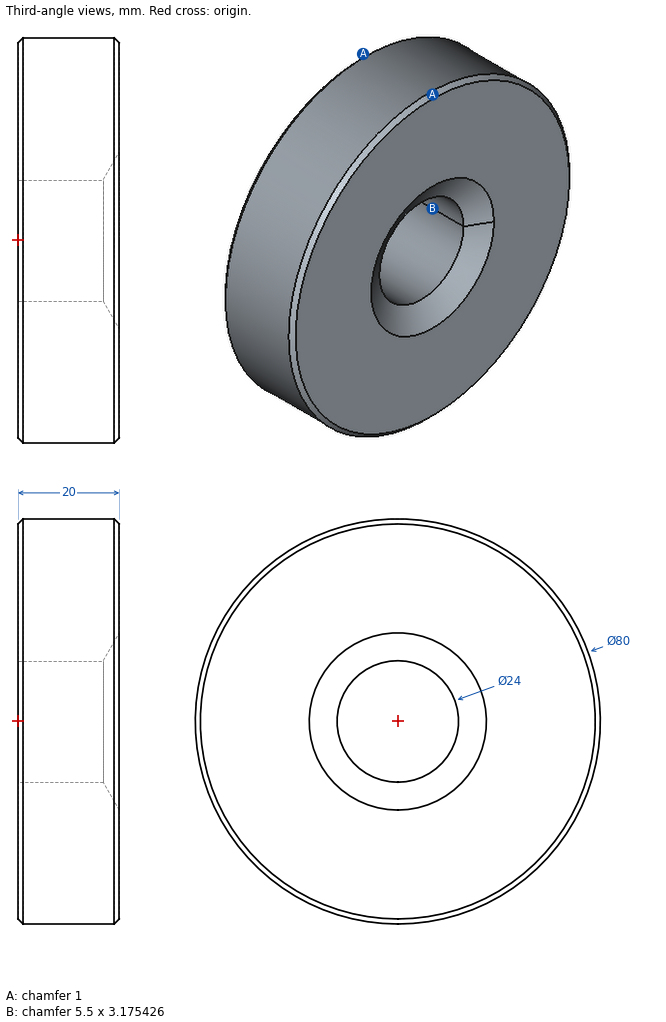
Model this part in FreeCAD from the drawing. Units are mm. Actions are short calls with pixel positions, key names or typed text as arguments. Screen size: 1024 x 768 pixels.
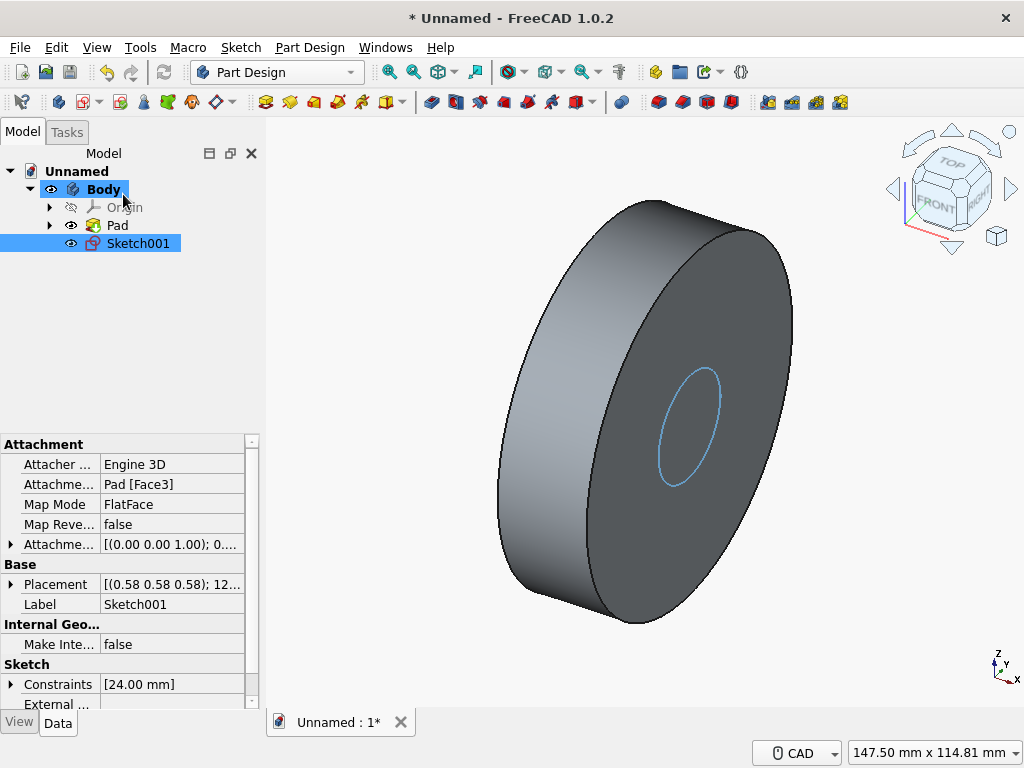
click(432, 102)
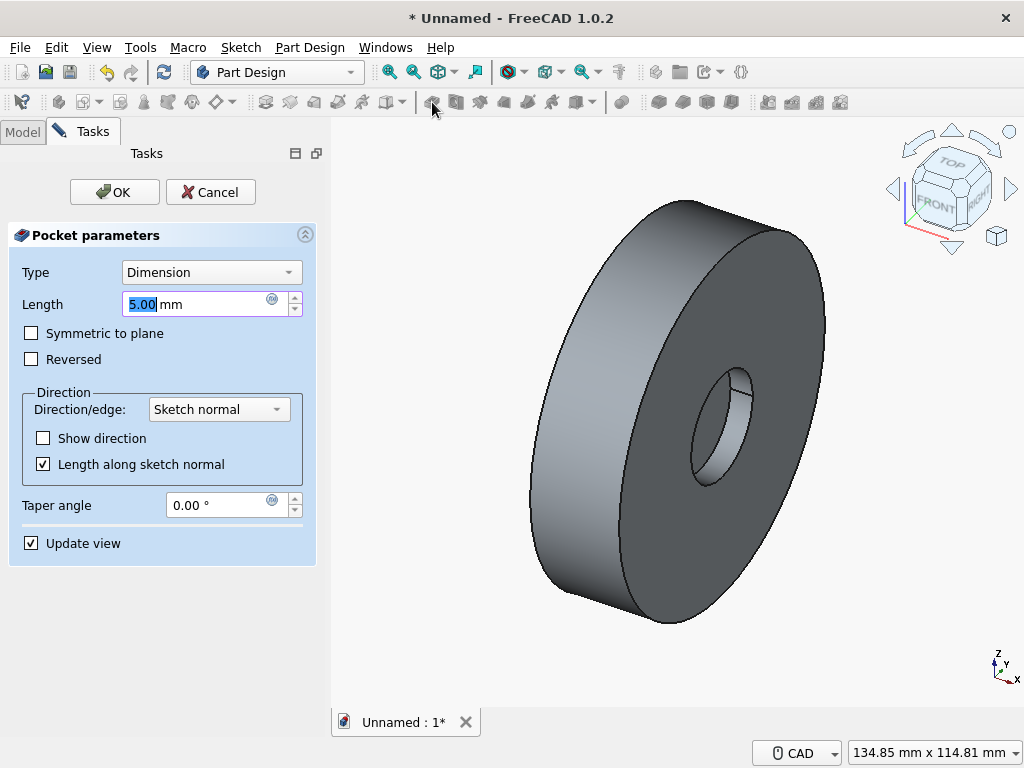
click(212, 272)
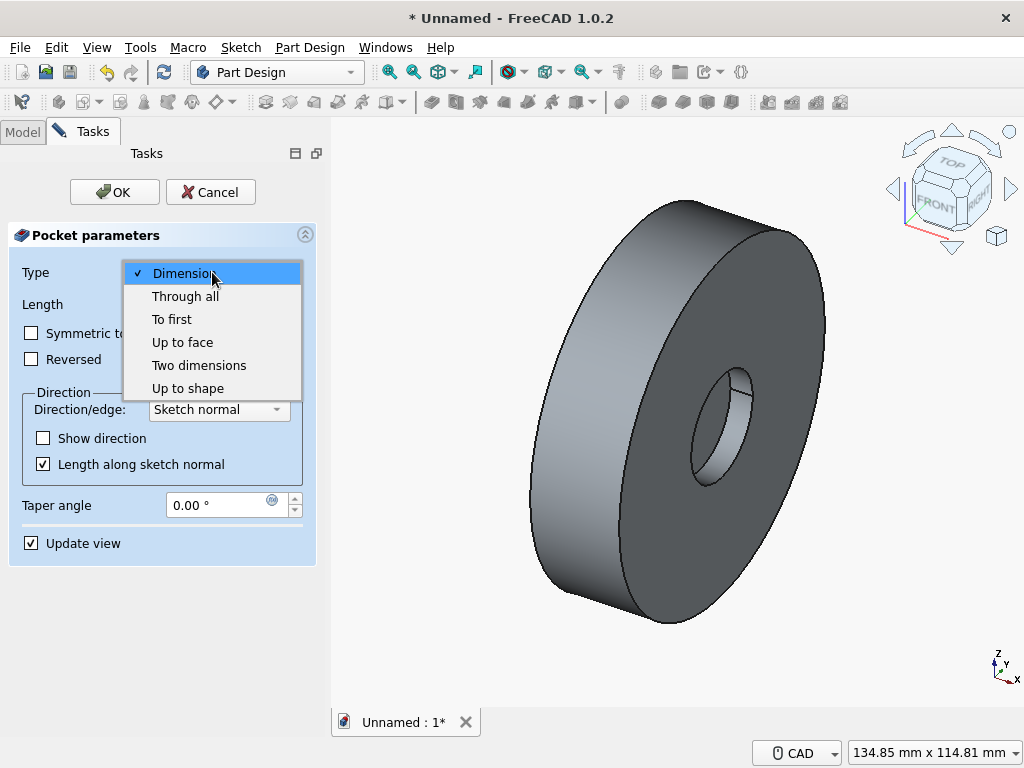
click(212, 296)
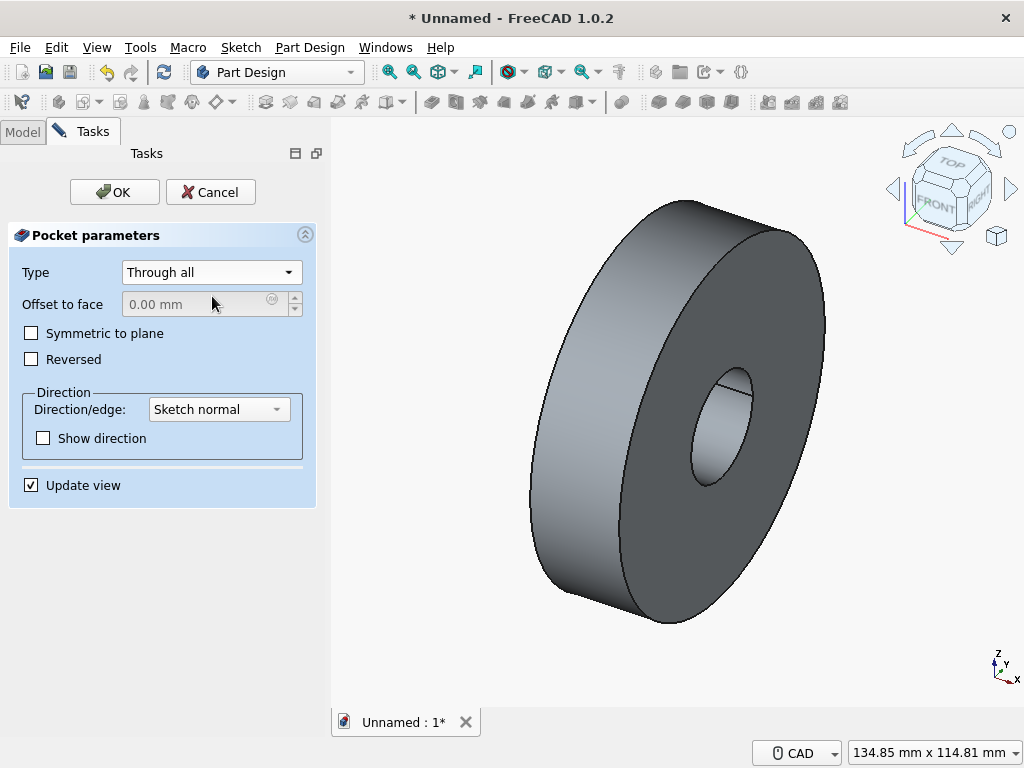
click(115, 192)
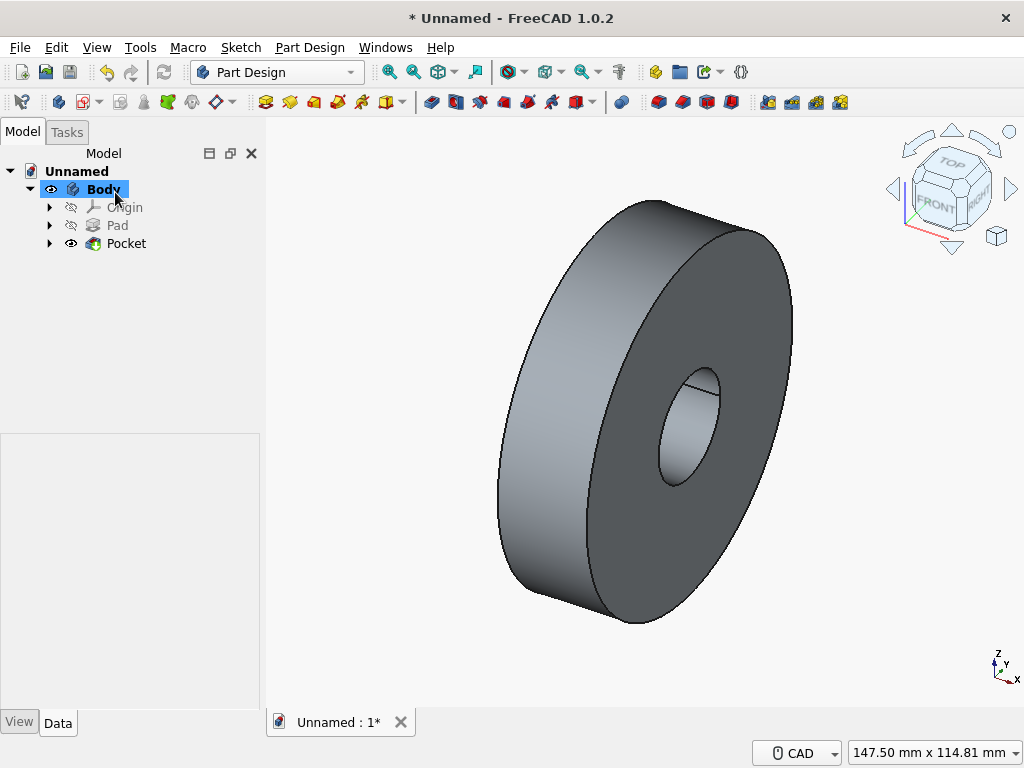
click(587, 528)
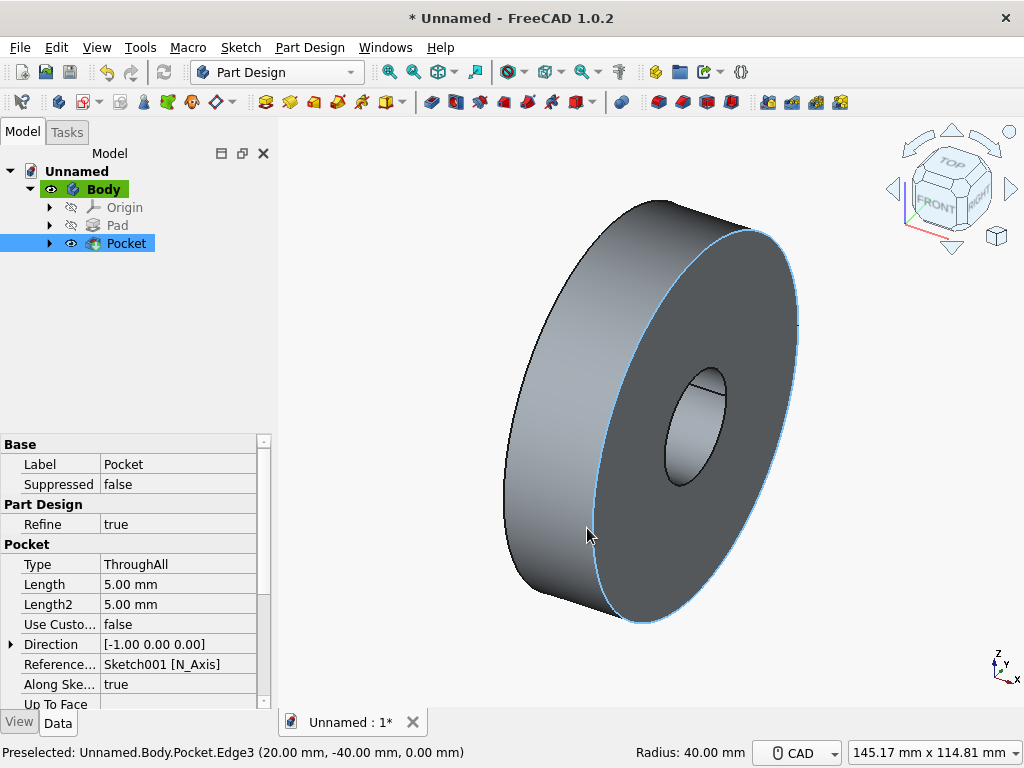
key(0)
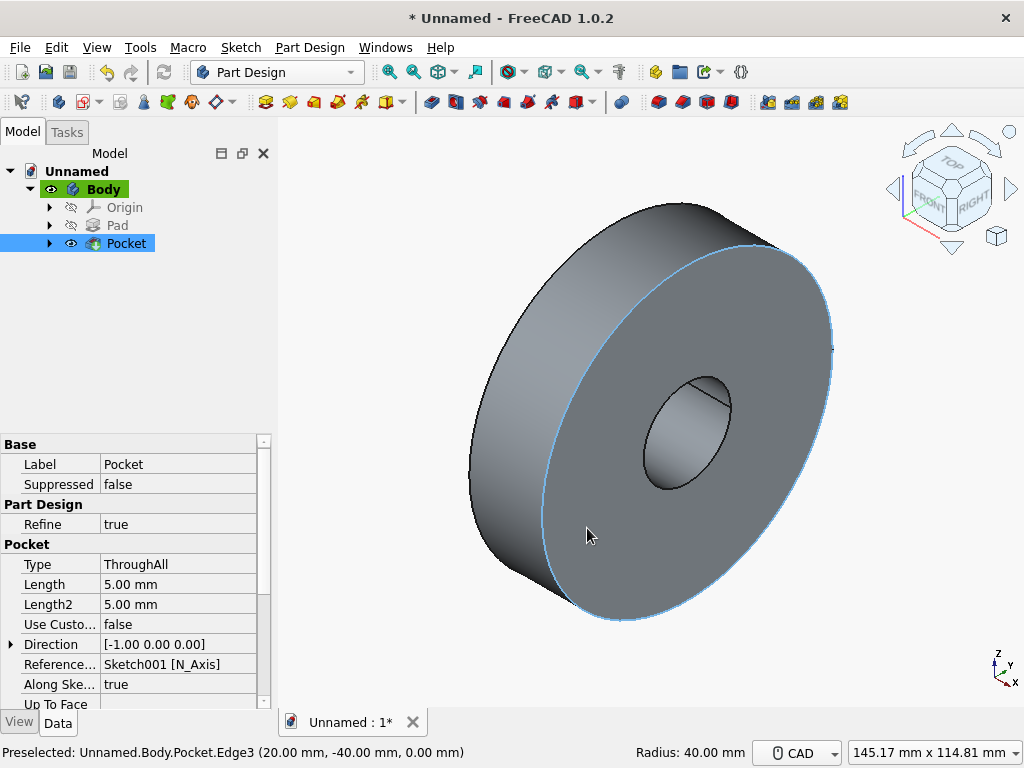
key(2)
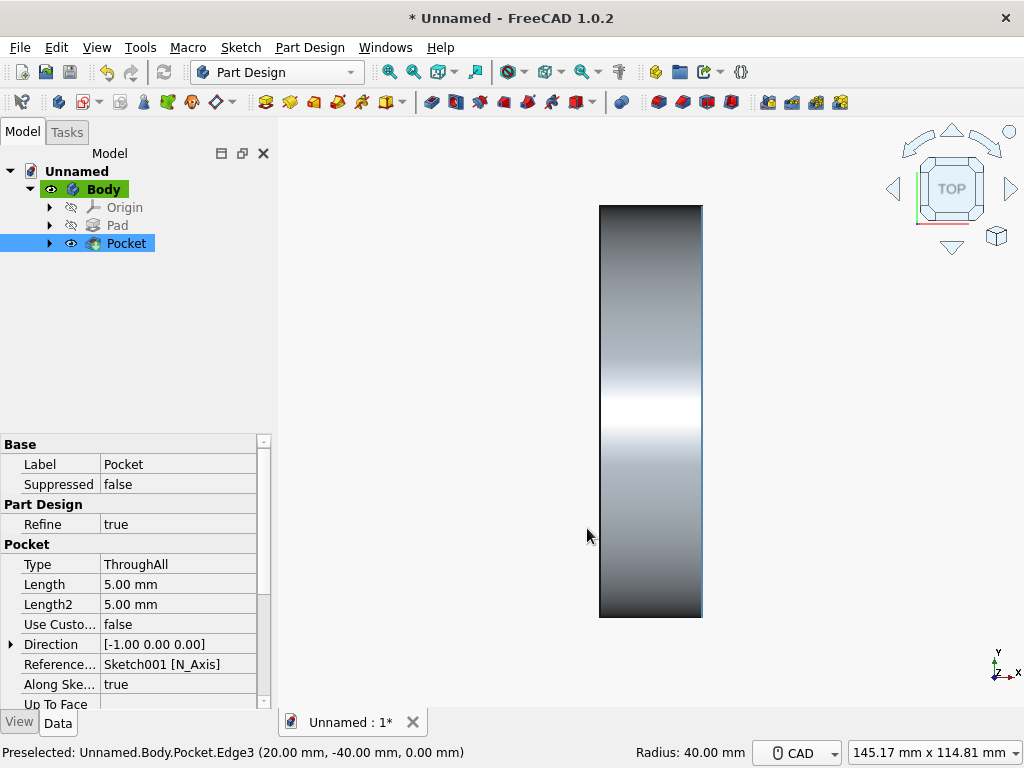
click(600, 577, ctrl)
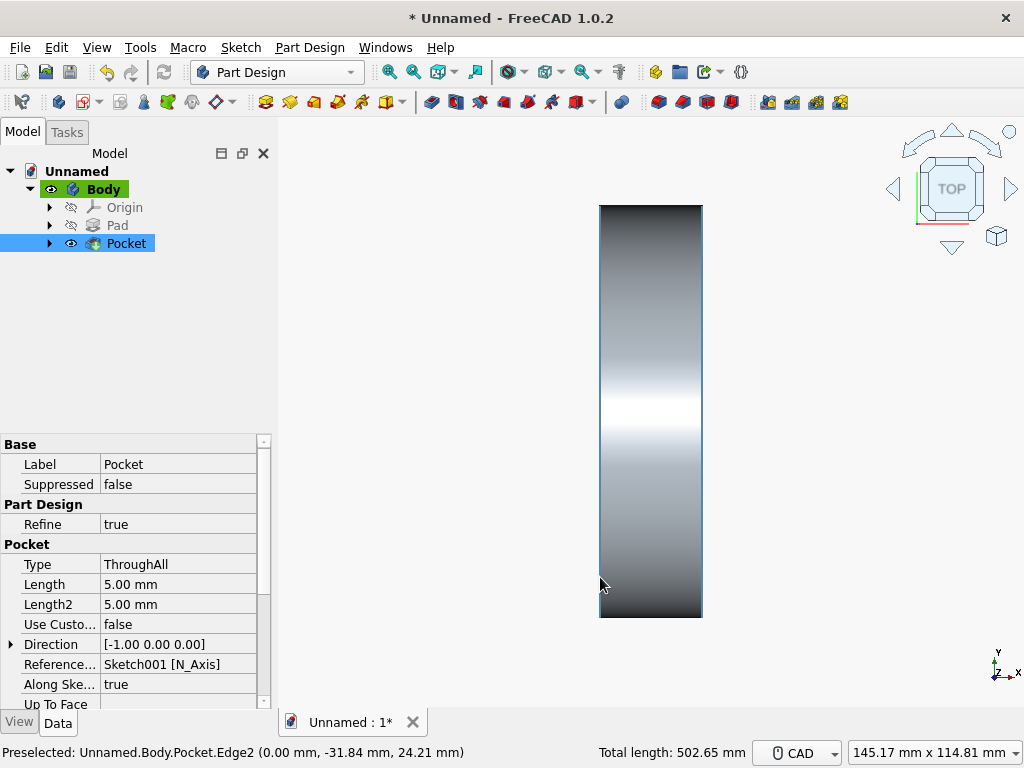
click(684, 102)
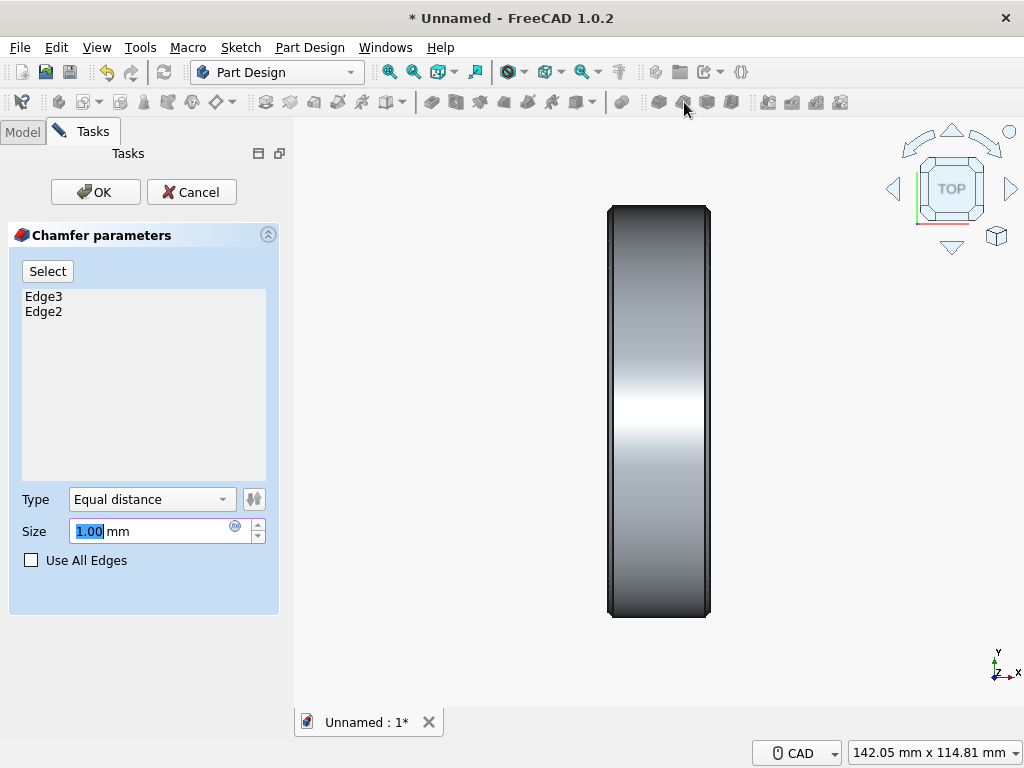
text(1)
key(Tab)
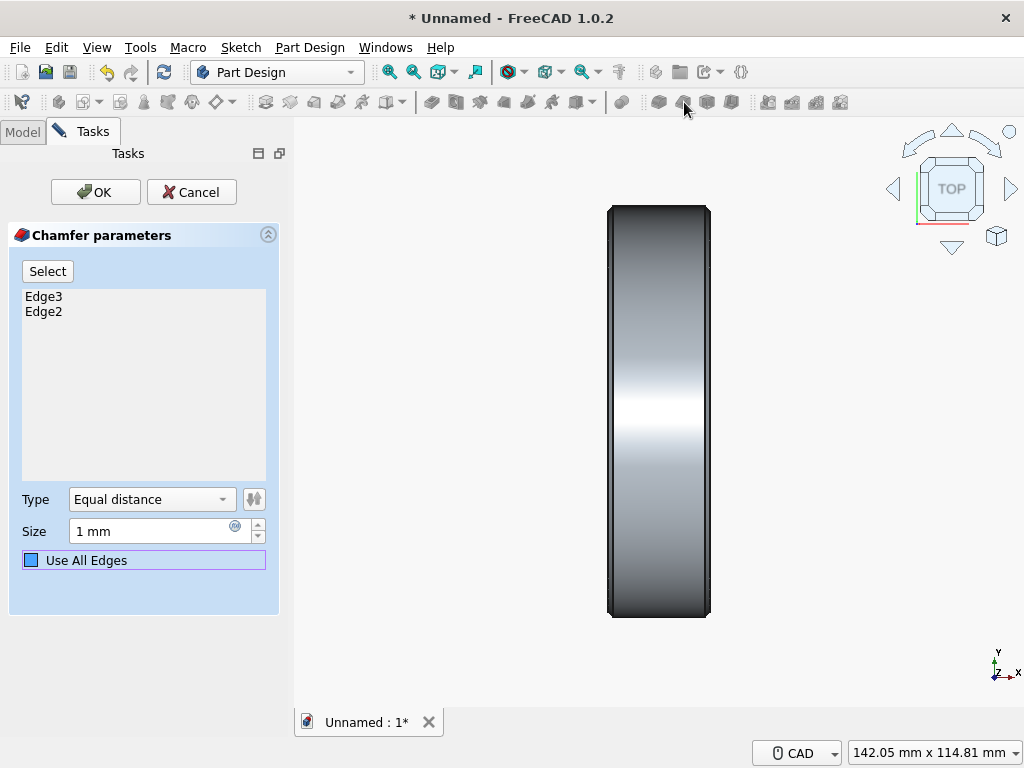
click(96, 192)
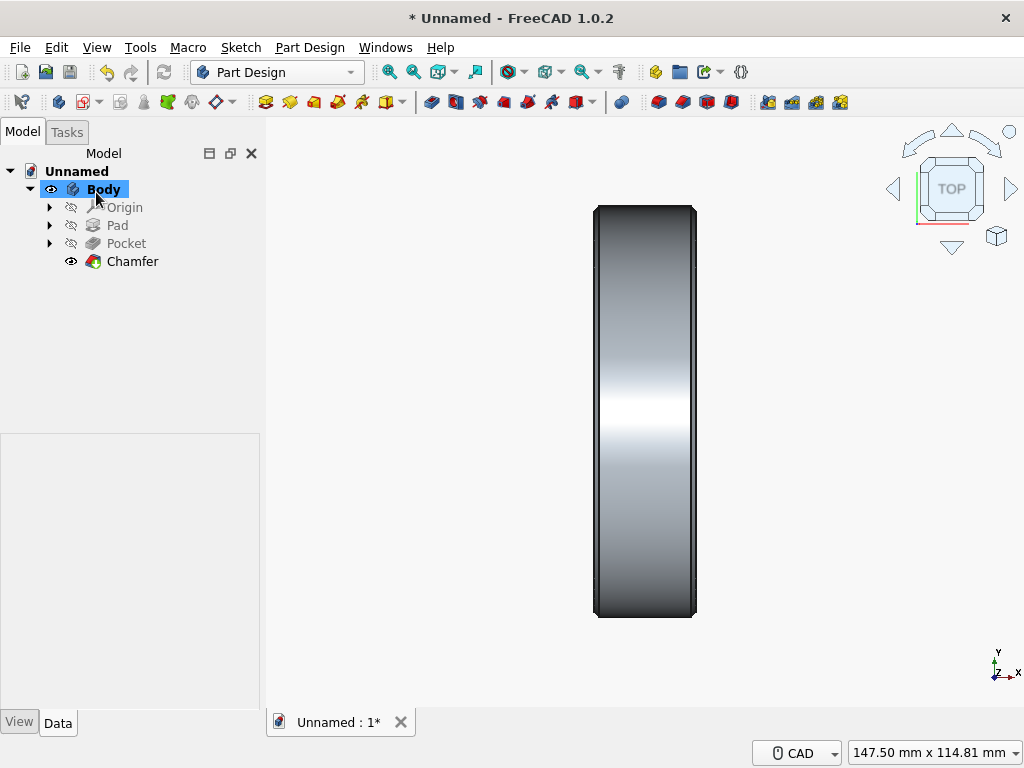
key(0)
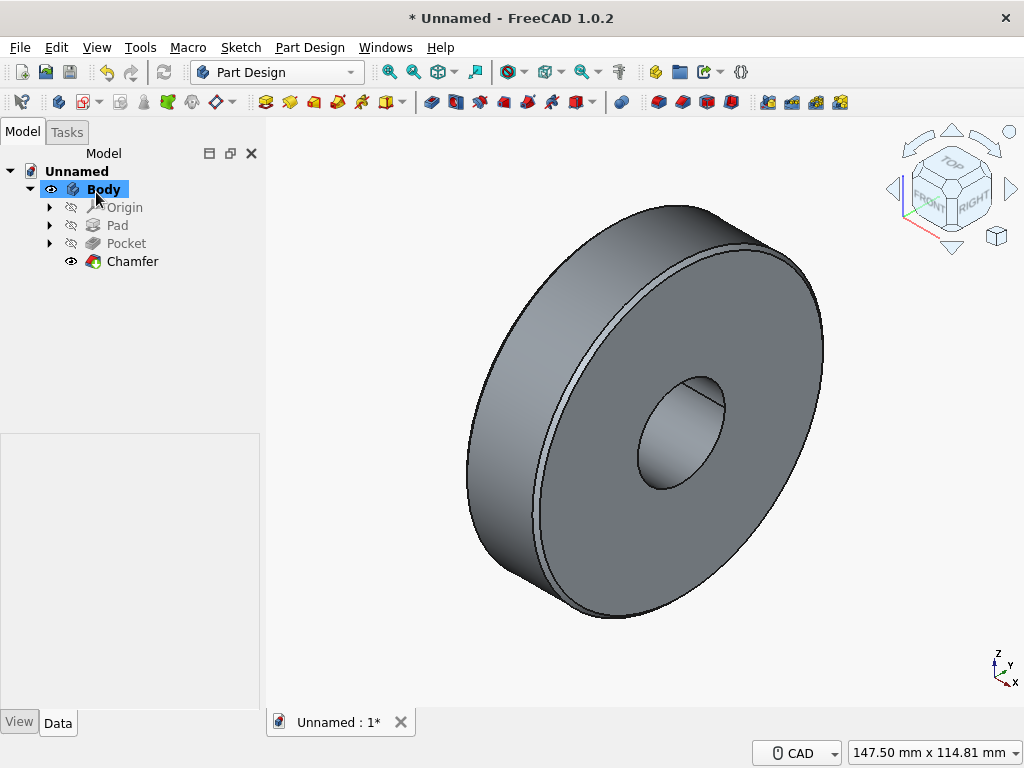
click(668, 488)